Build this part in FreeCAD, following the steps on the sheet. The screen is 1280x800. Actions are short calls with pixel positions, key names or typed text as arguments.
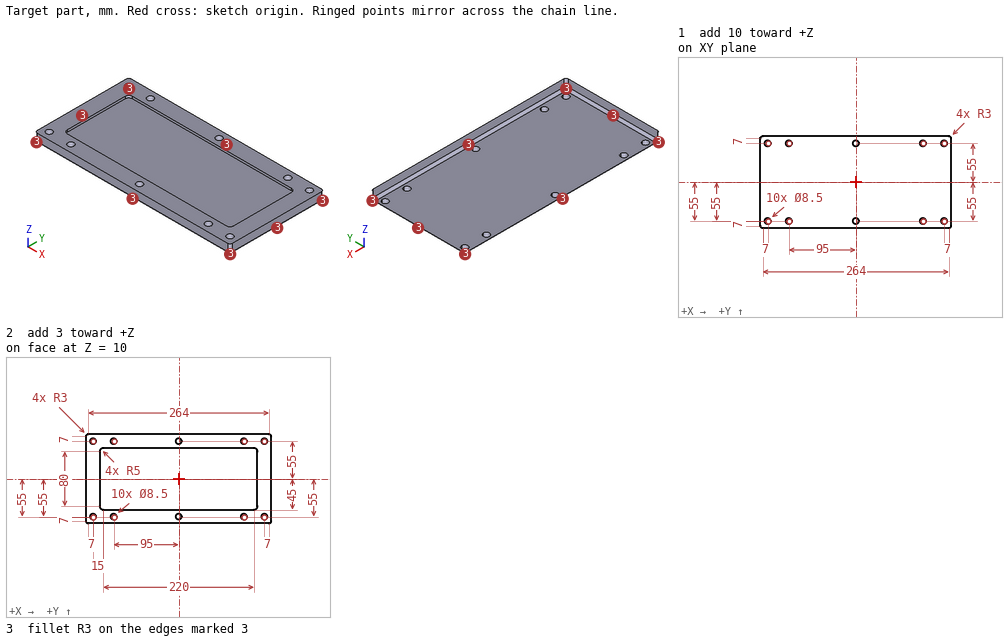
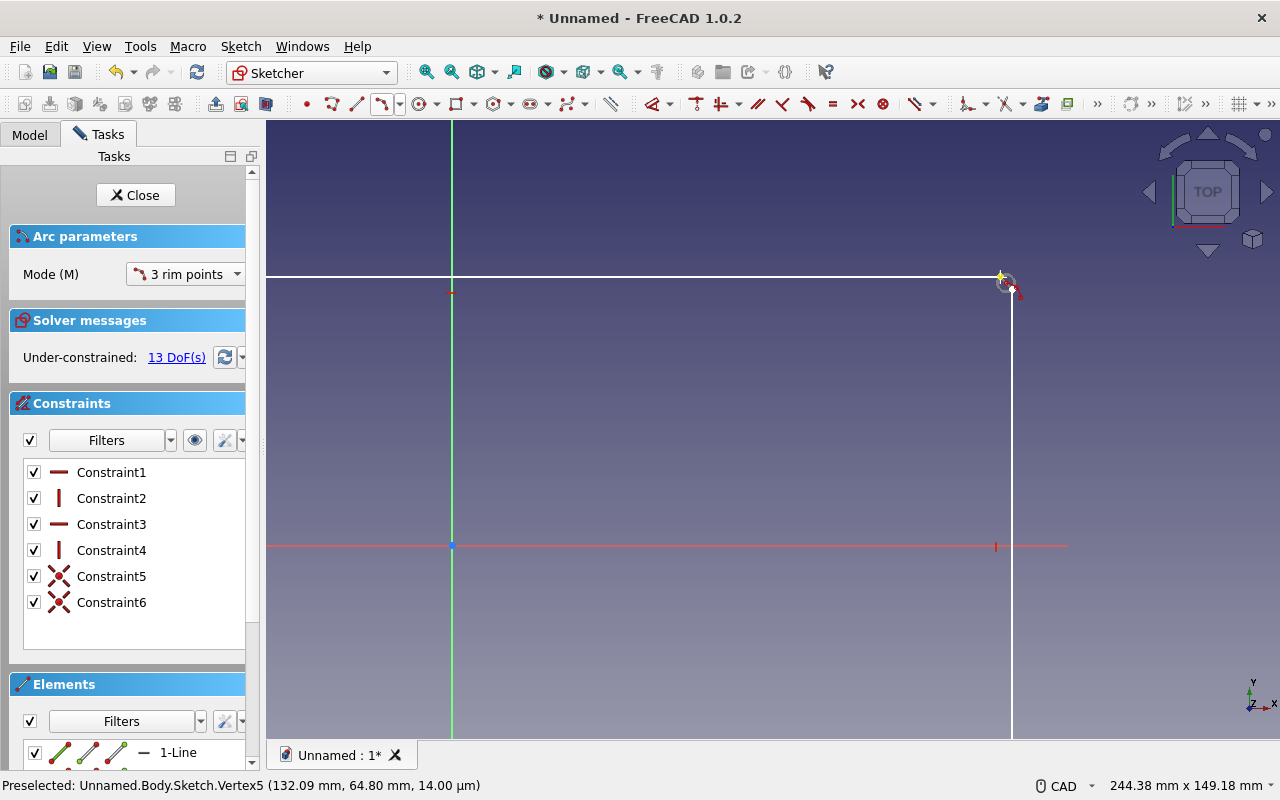
scroll(1009, 280, up, 8)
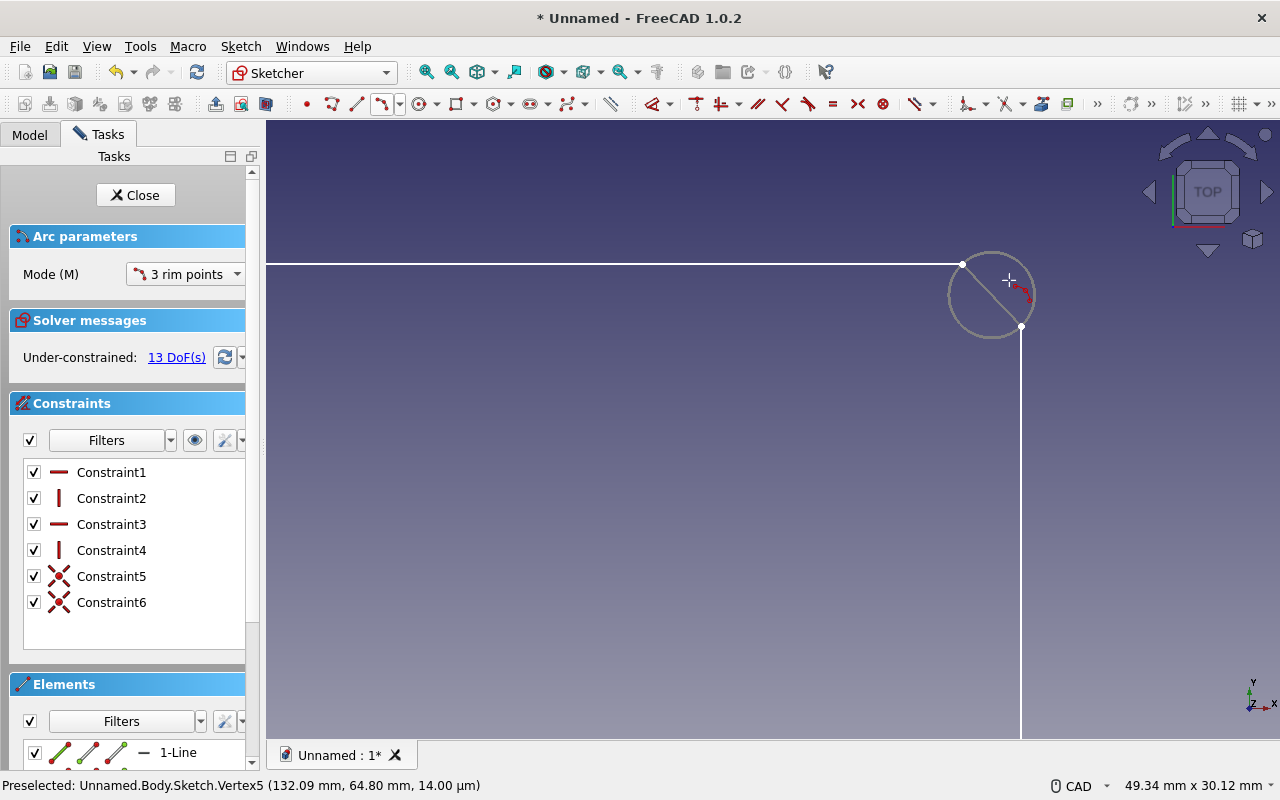
click(1004, 278)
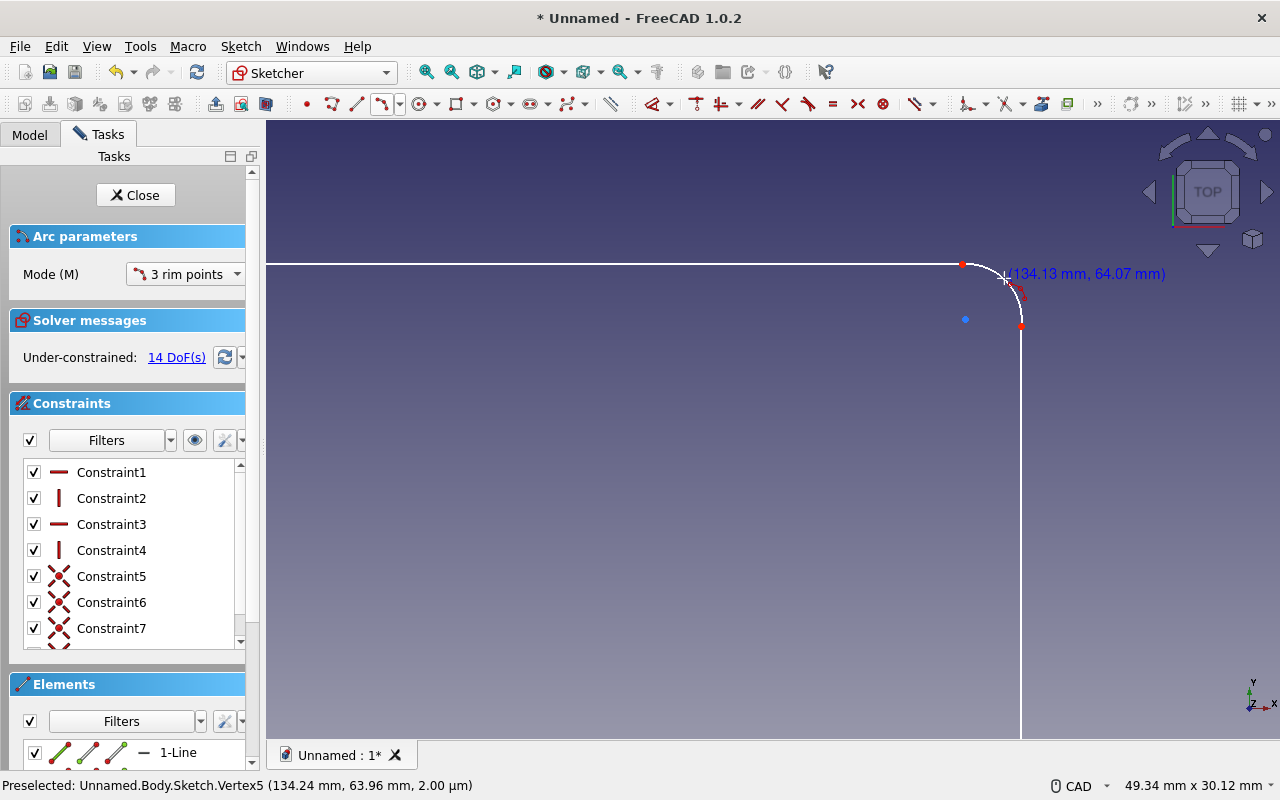
scroll(1011, 284, down, 11)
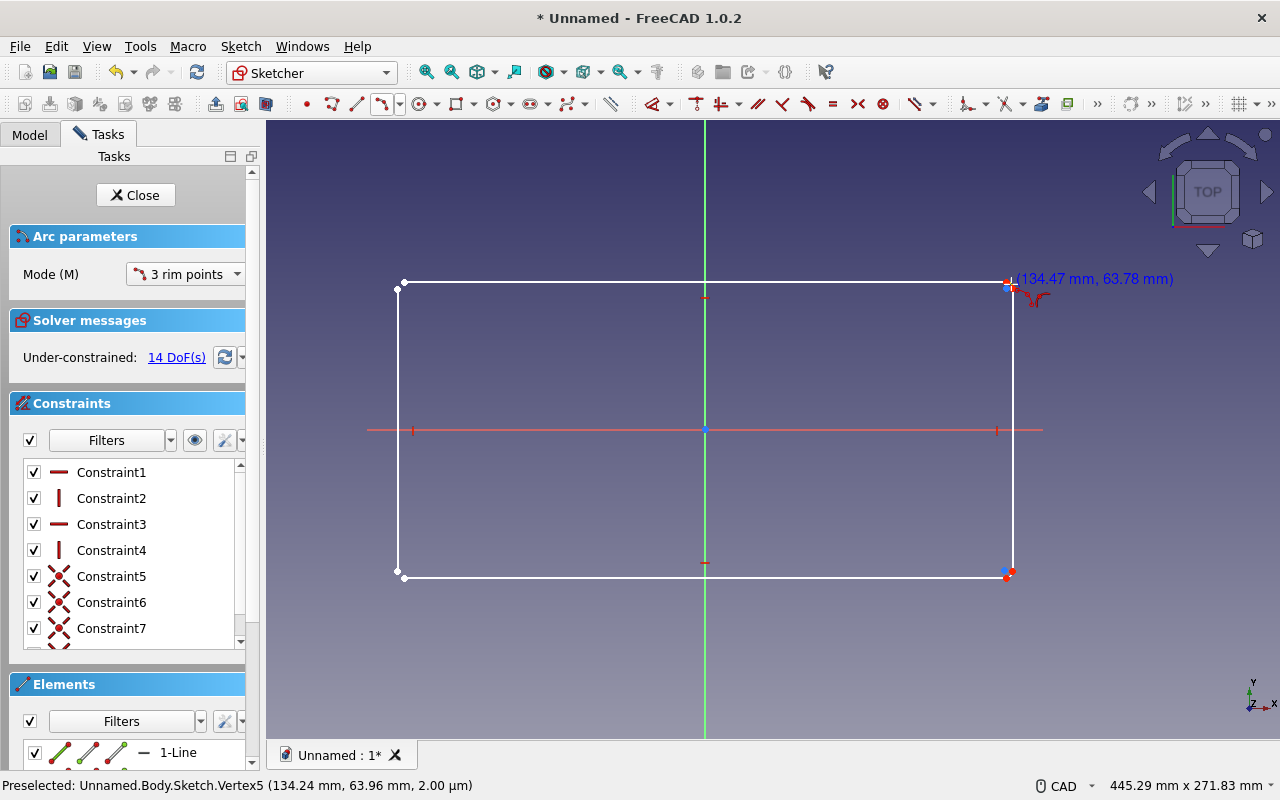
scroll(405, 282, up, 3)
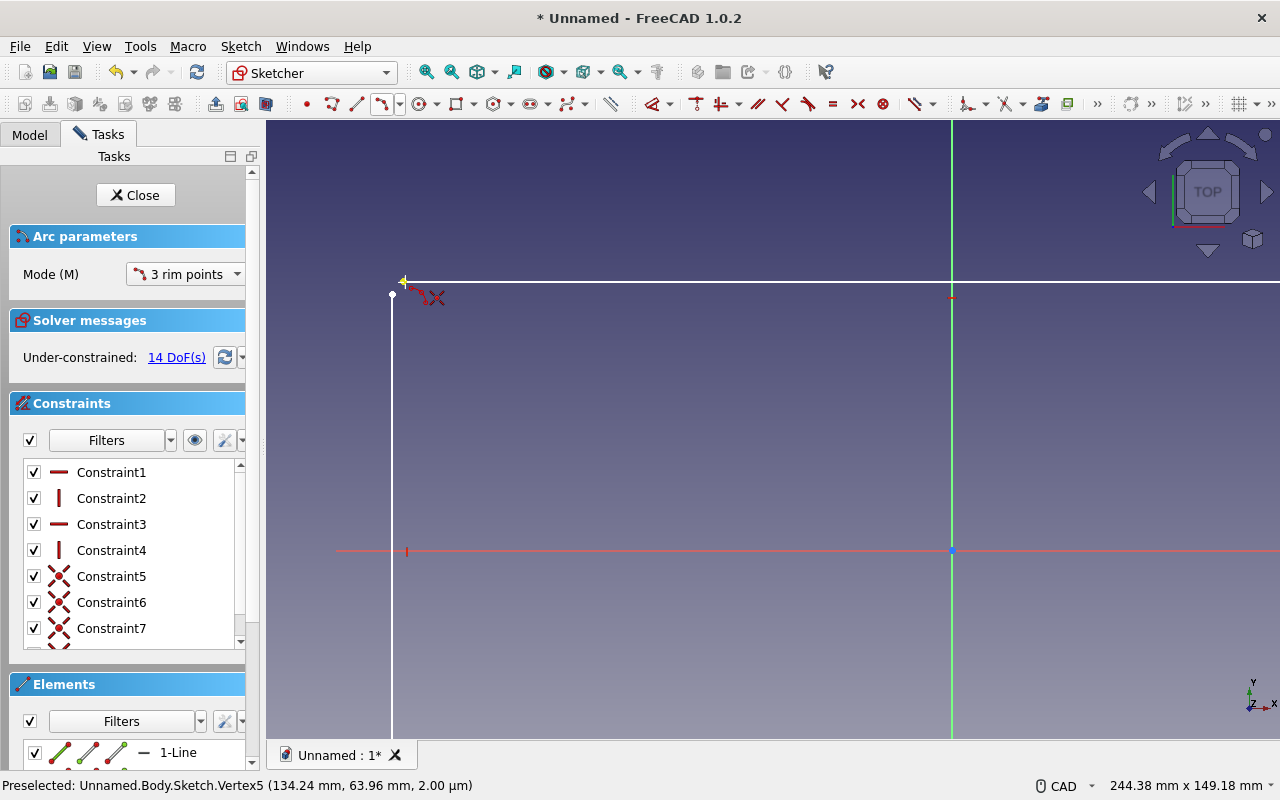
click(404, 282)
click(392, 295)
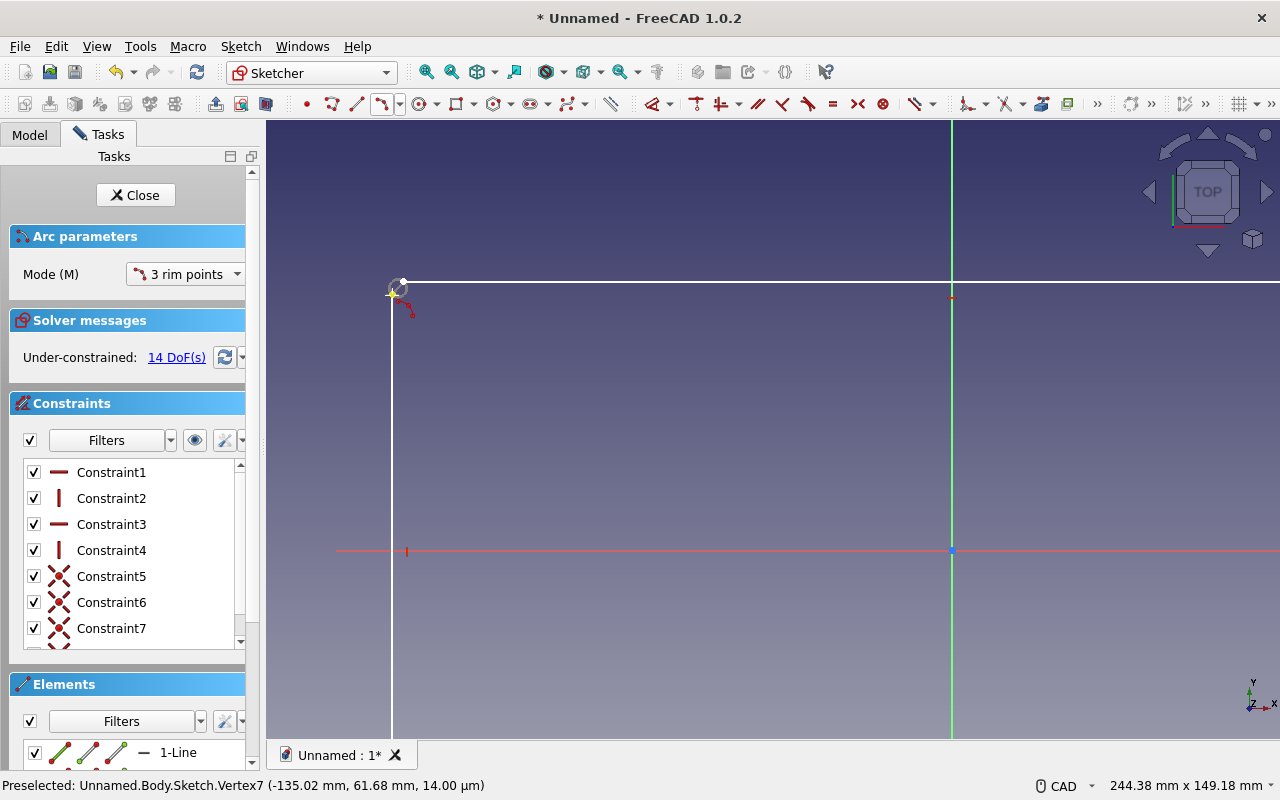
scroll(396, 285, up, 8)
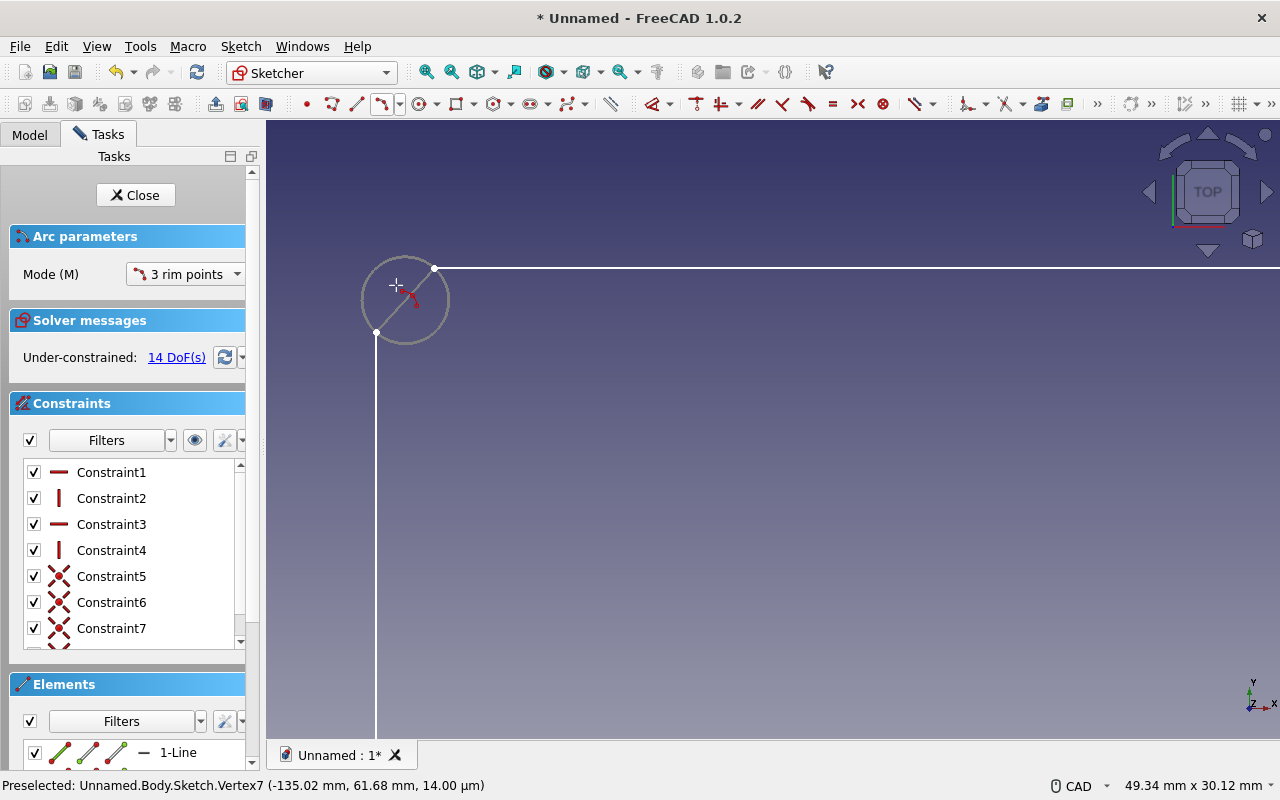
click(395, 282)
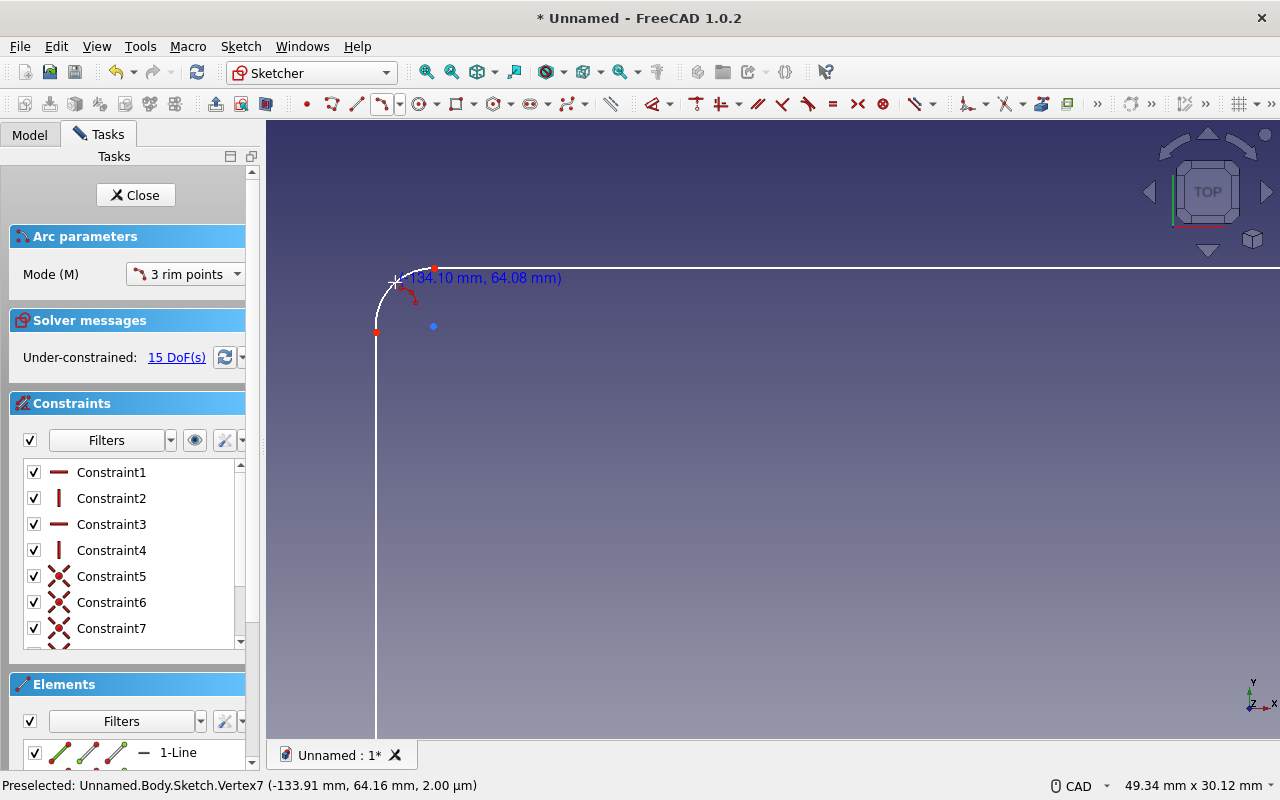
scroll(400, 284, down, 11)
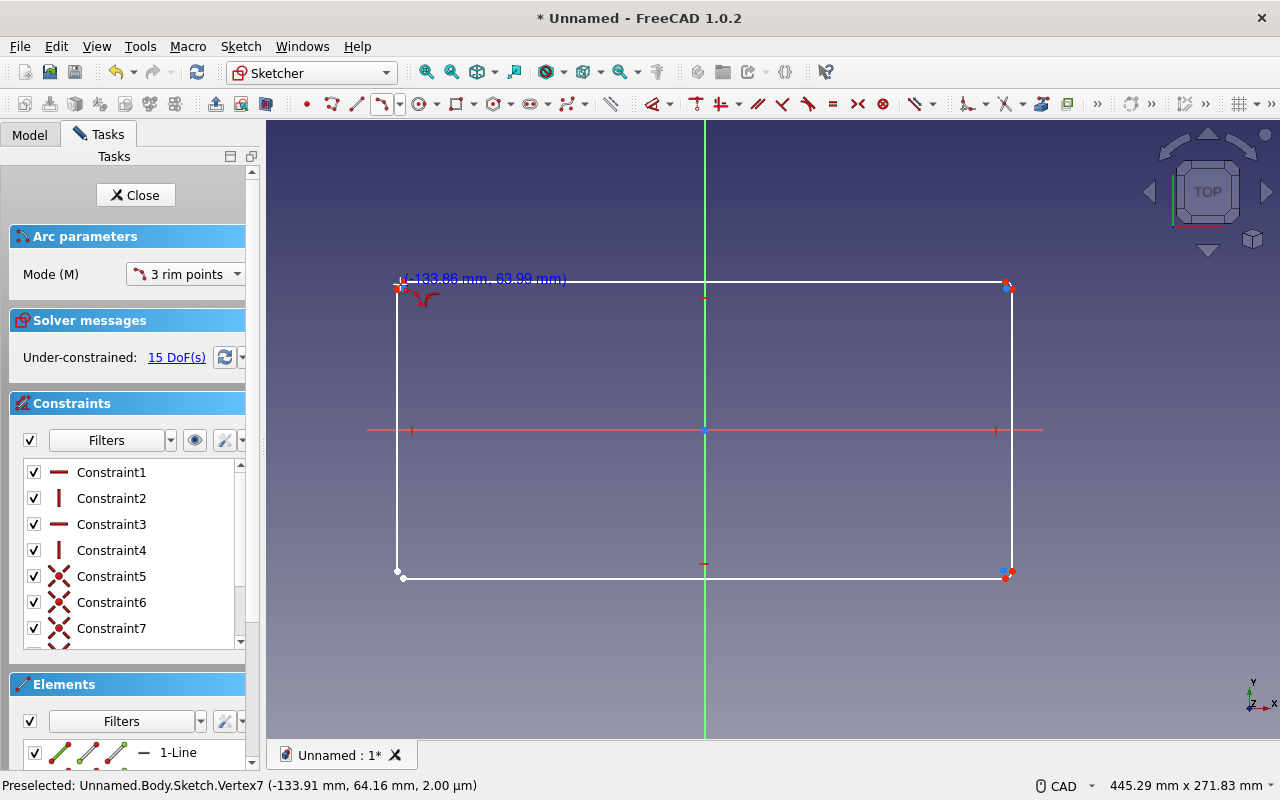
scroll(398, 571, up, 3)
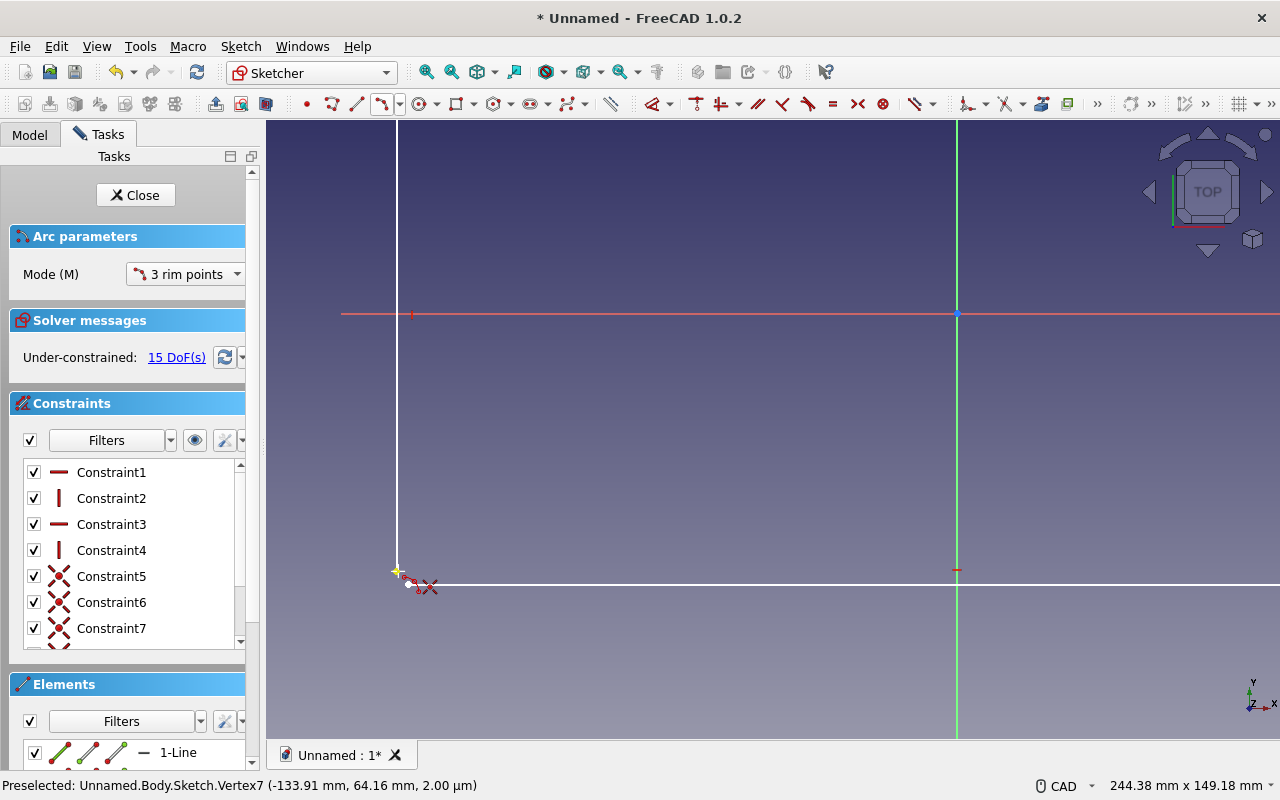
click(397, 572)
click(409, 585)